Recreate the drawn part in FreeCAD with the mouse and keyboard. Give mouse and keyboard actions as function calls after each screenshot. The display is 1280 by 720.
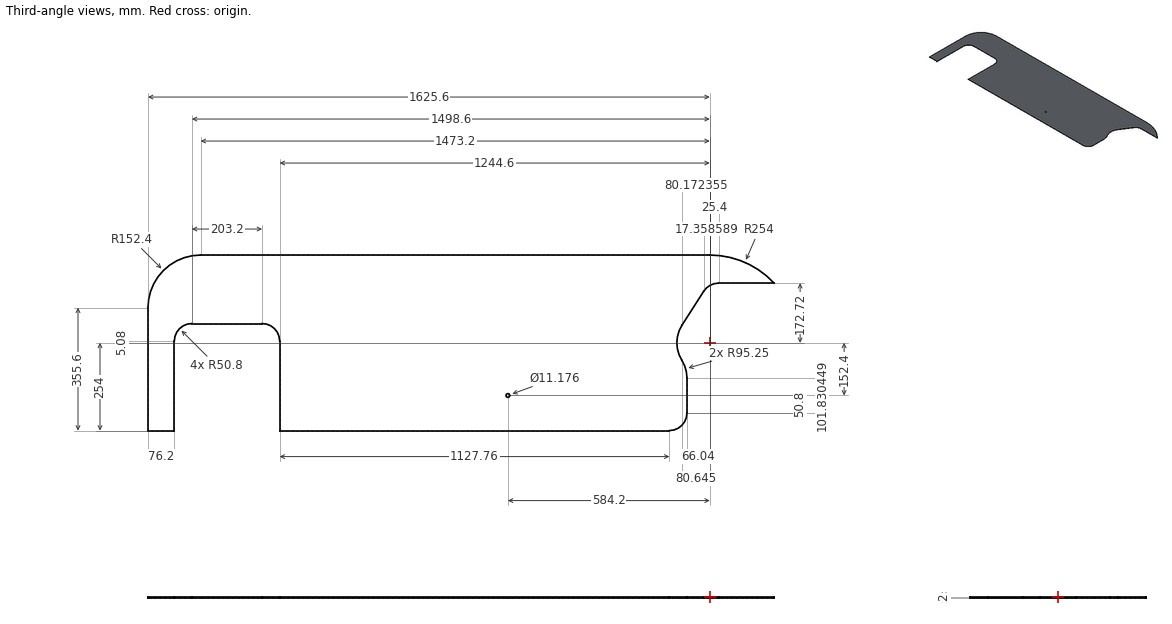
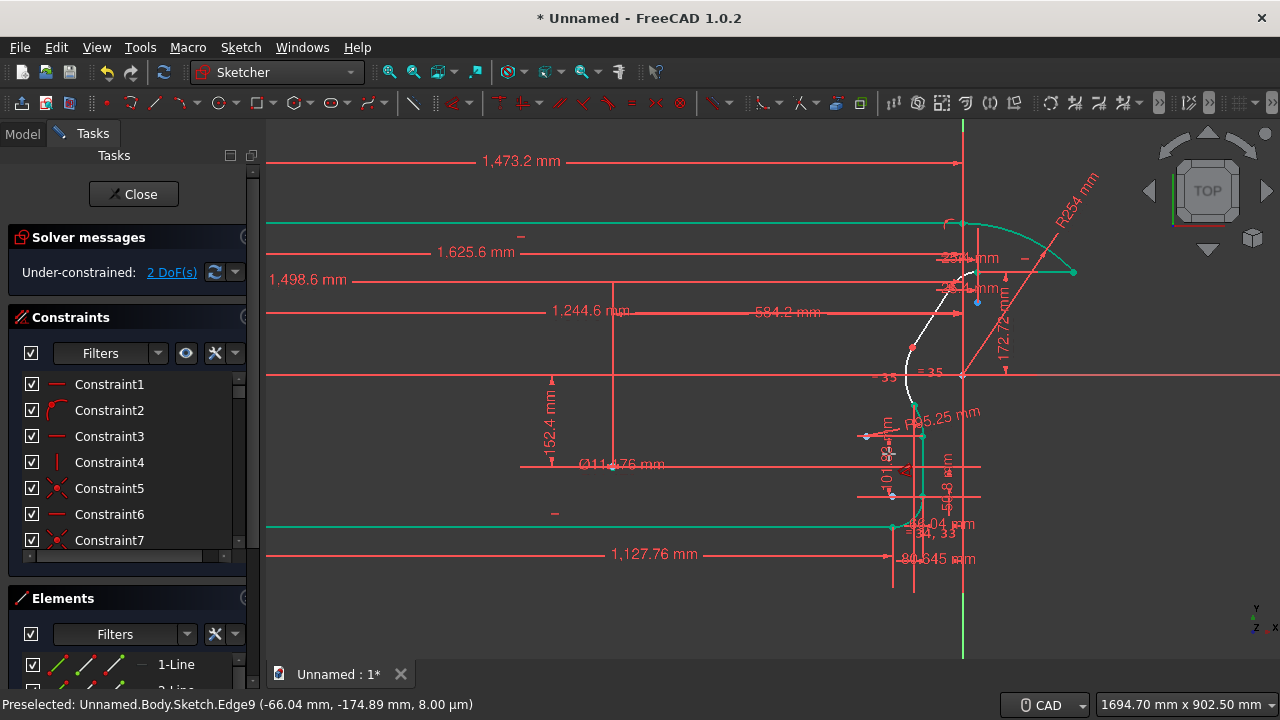
click(913, 347)
click(938, 193)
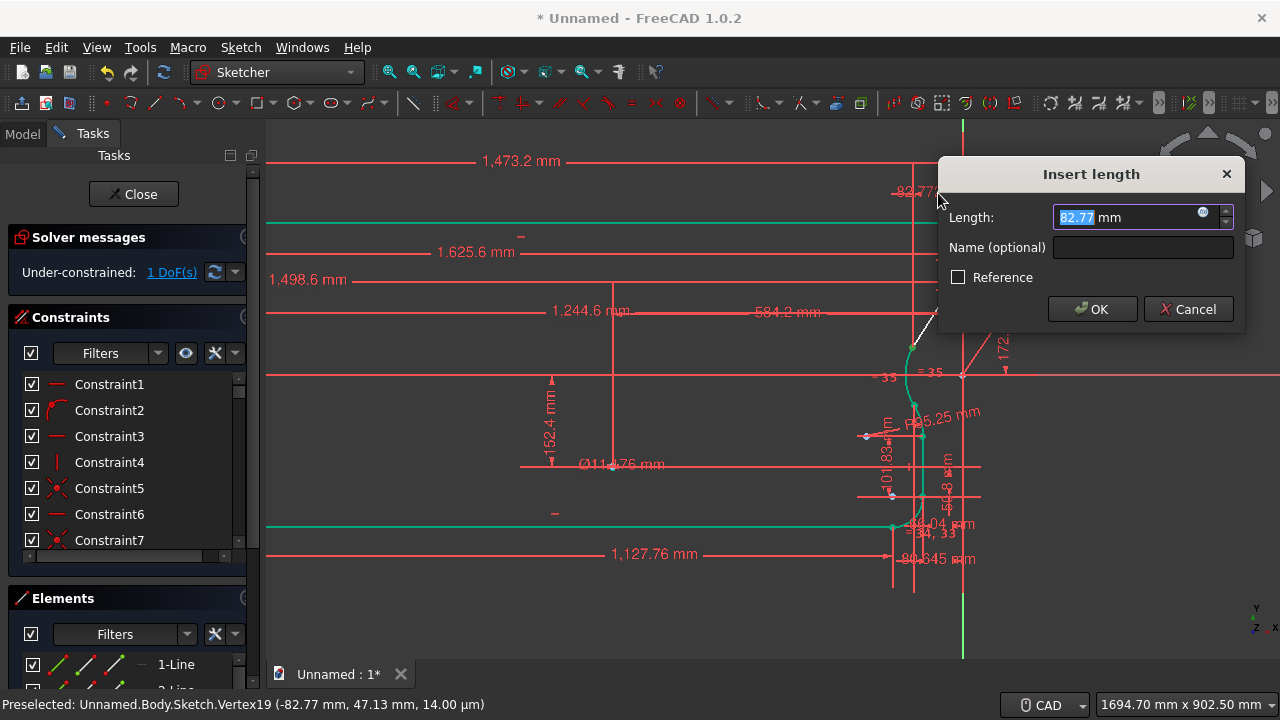
text(80.172355)
key(Return)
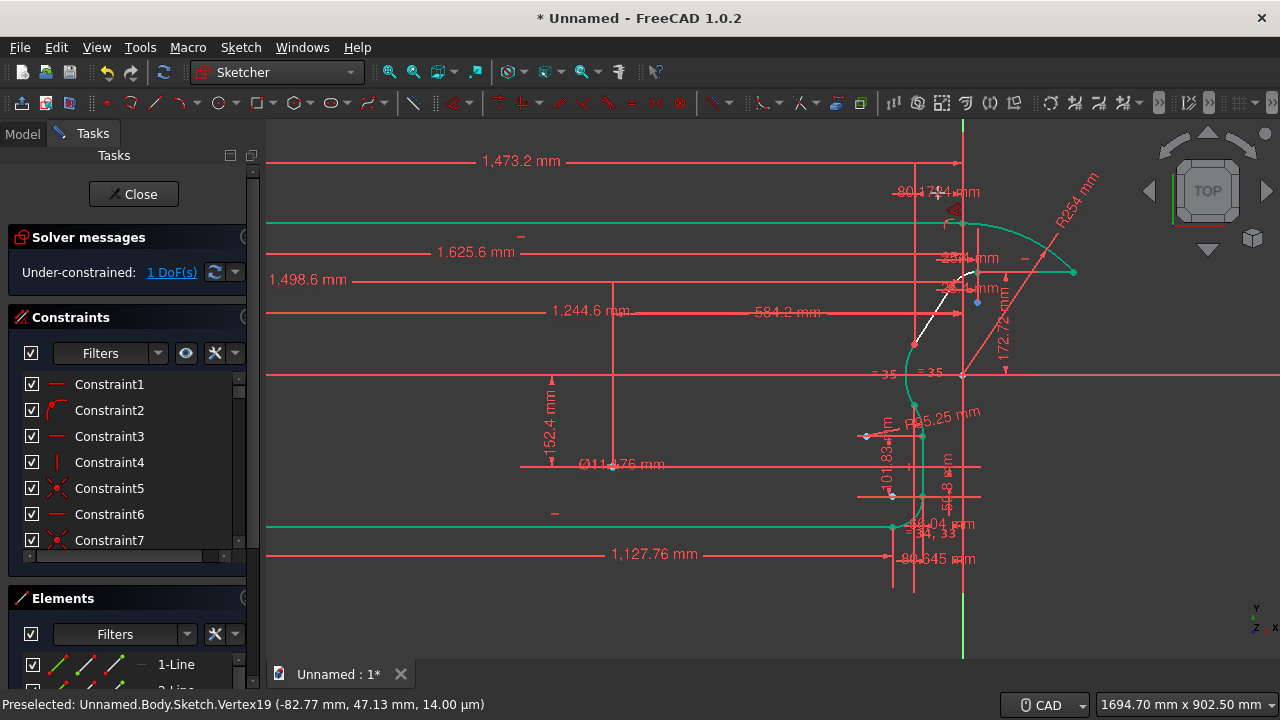
scroll(952, 286, up, 7)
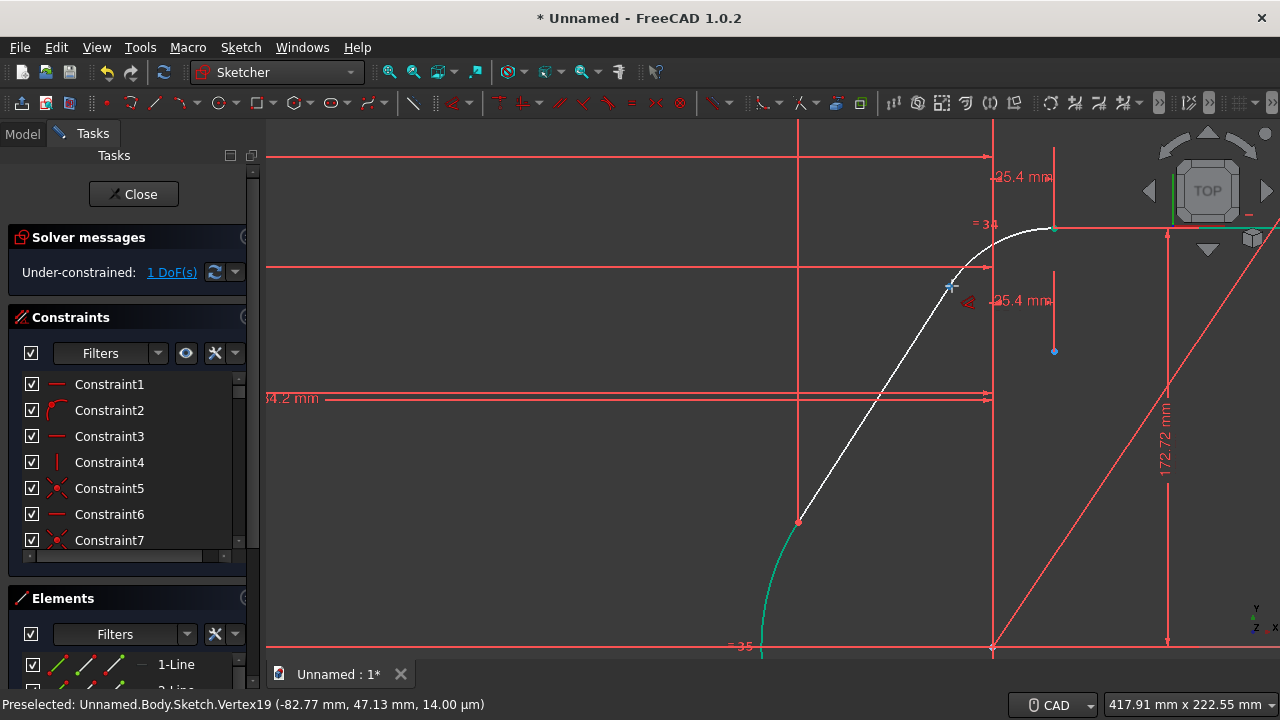
click(950, 286)
click(956, 252)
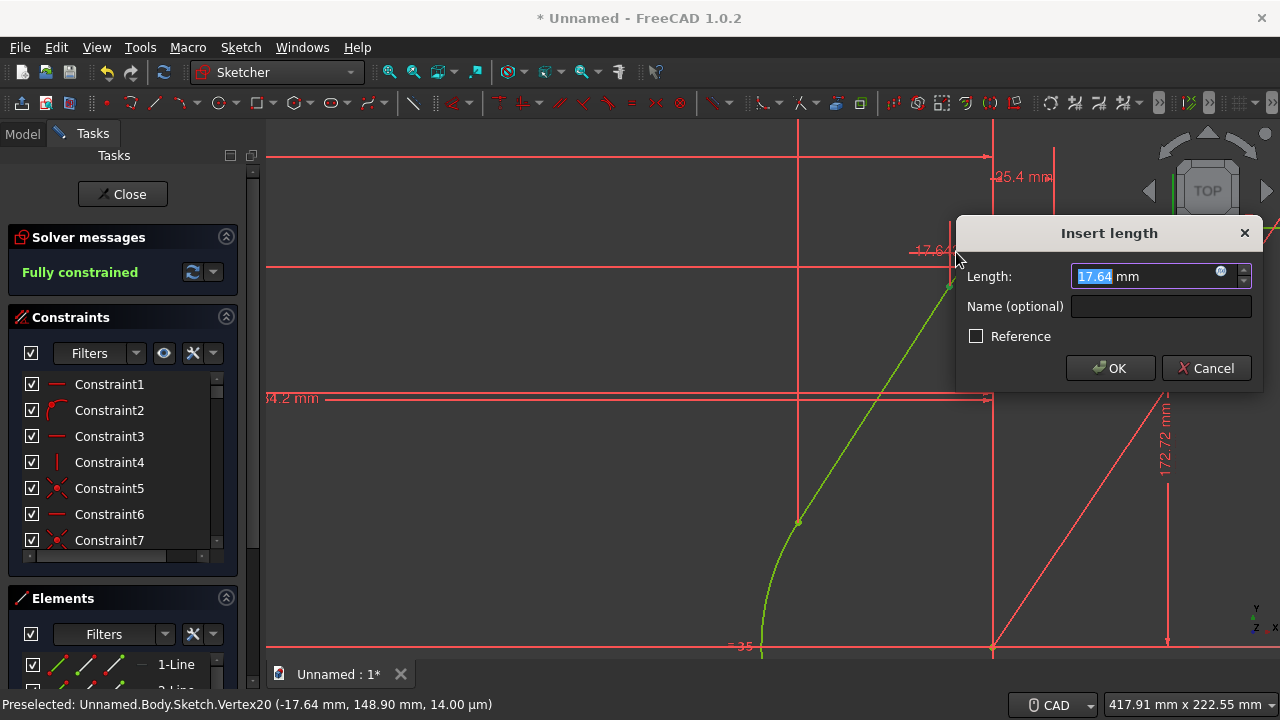
text(17.358589)
key(Return)
key(Escape)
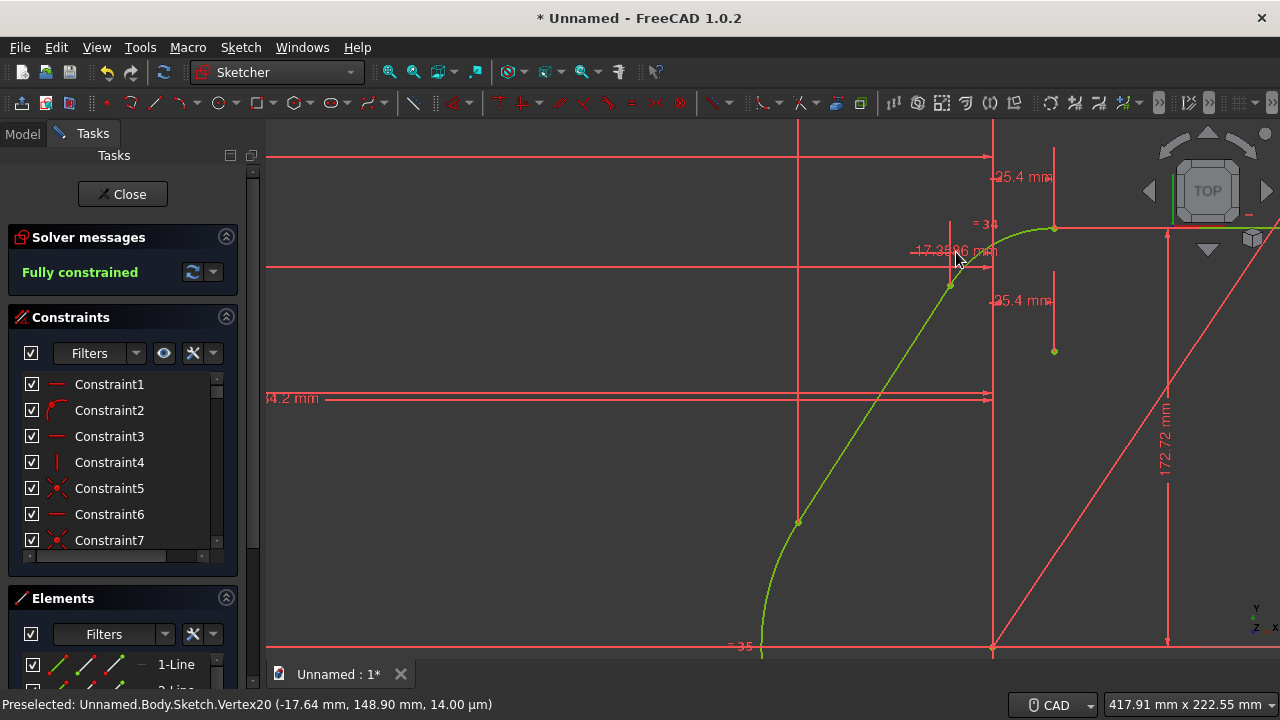
click(123, 194)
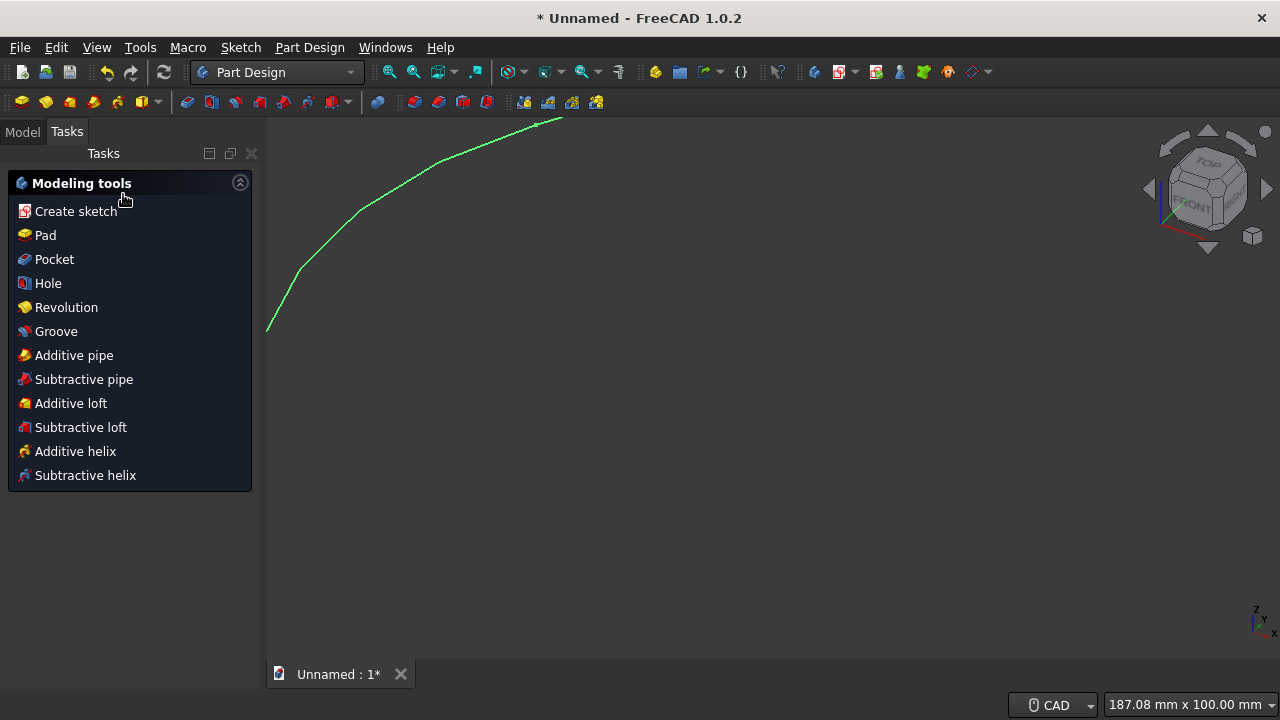
click(22, 102)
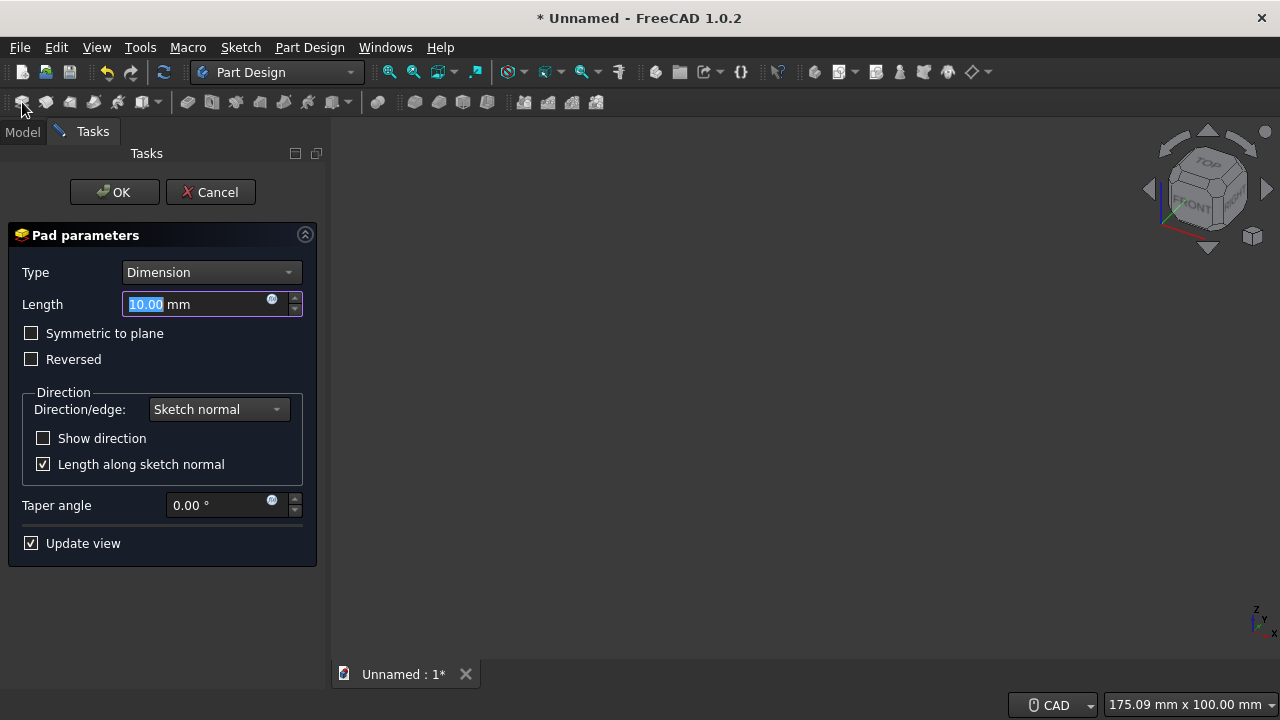
text(2)
key(Tab)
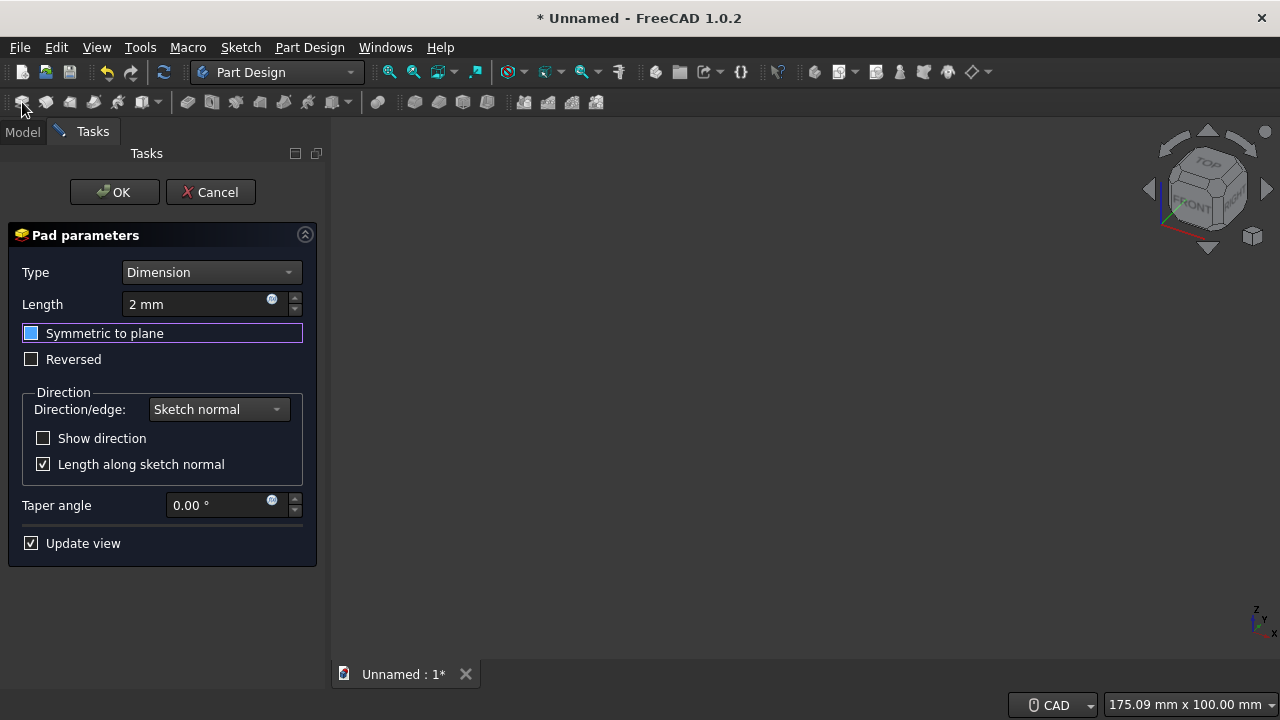
click(30, 333)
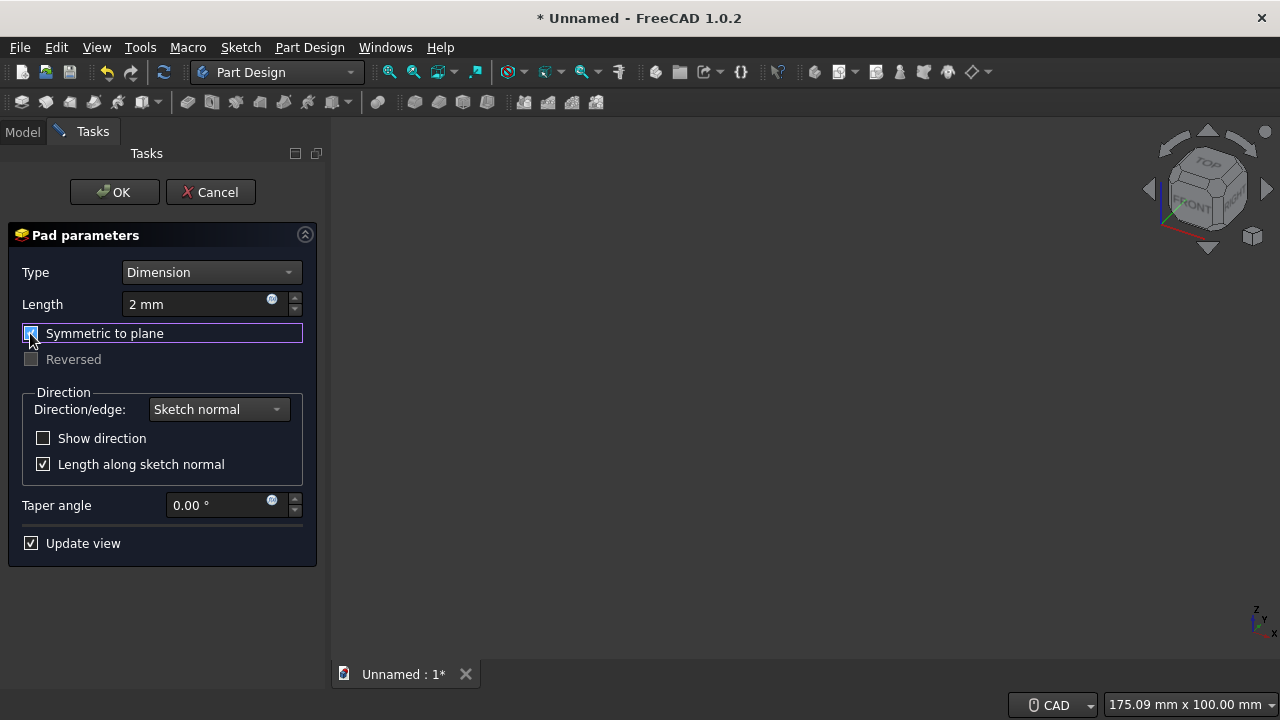
click(115, 192)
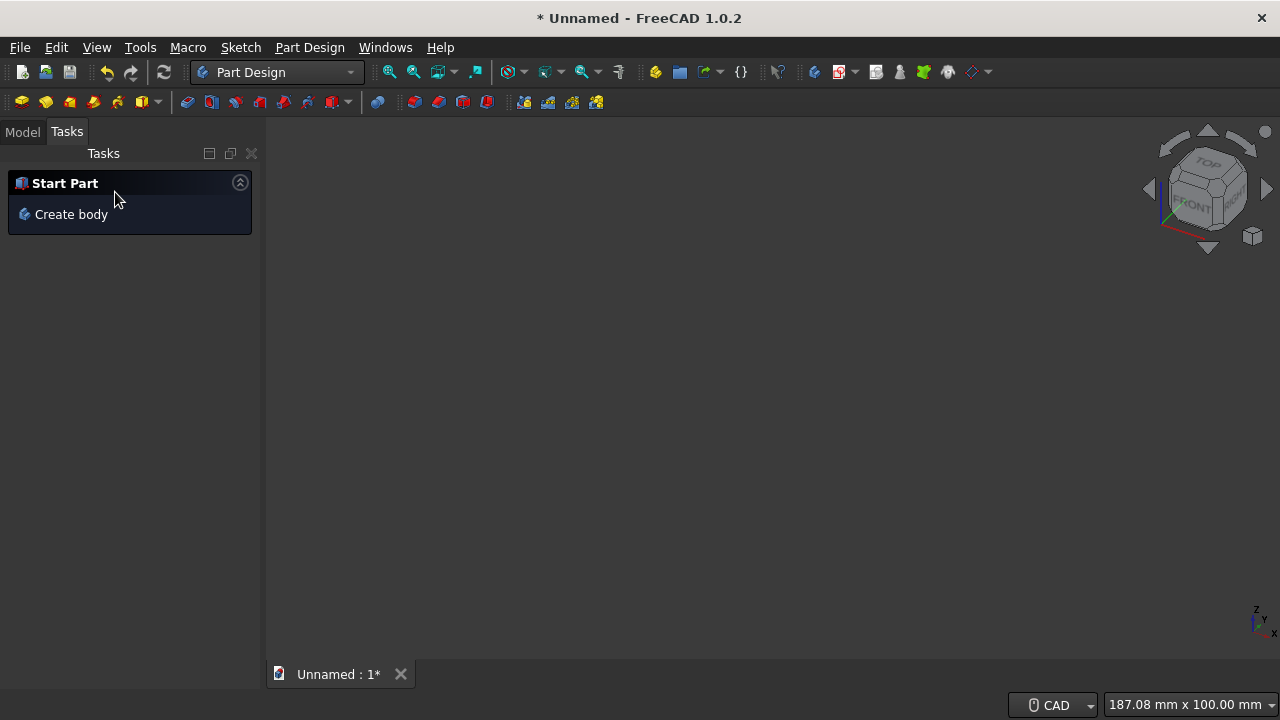
key(0)